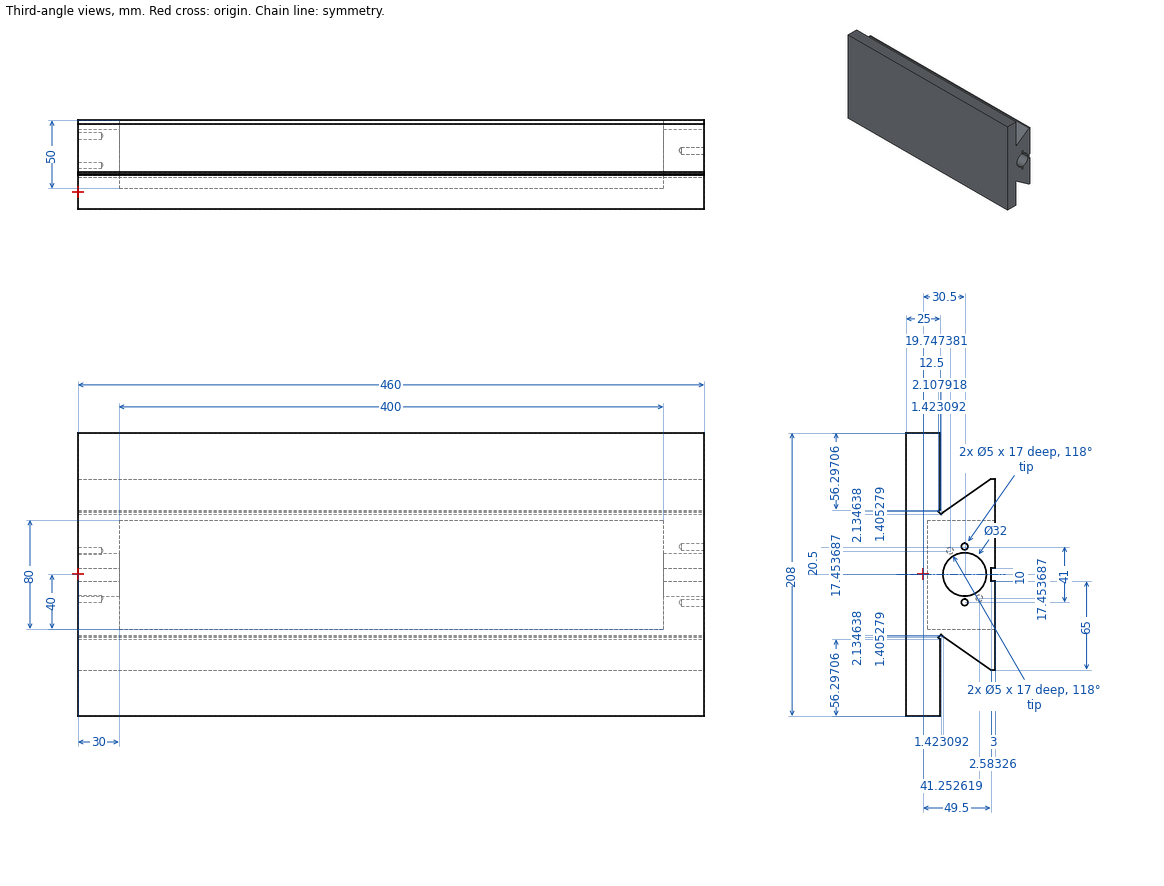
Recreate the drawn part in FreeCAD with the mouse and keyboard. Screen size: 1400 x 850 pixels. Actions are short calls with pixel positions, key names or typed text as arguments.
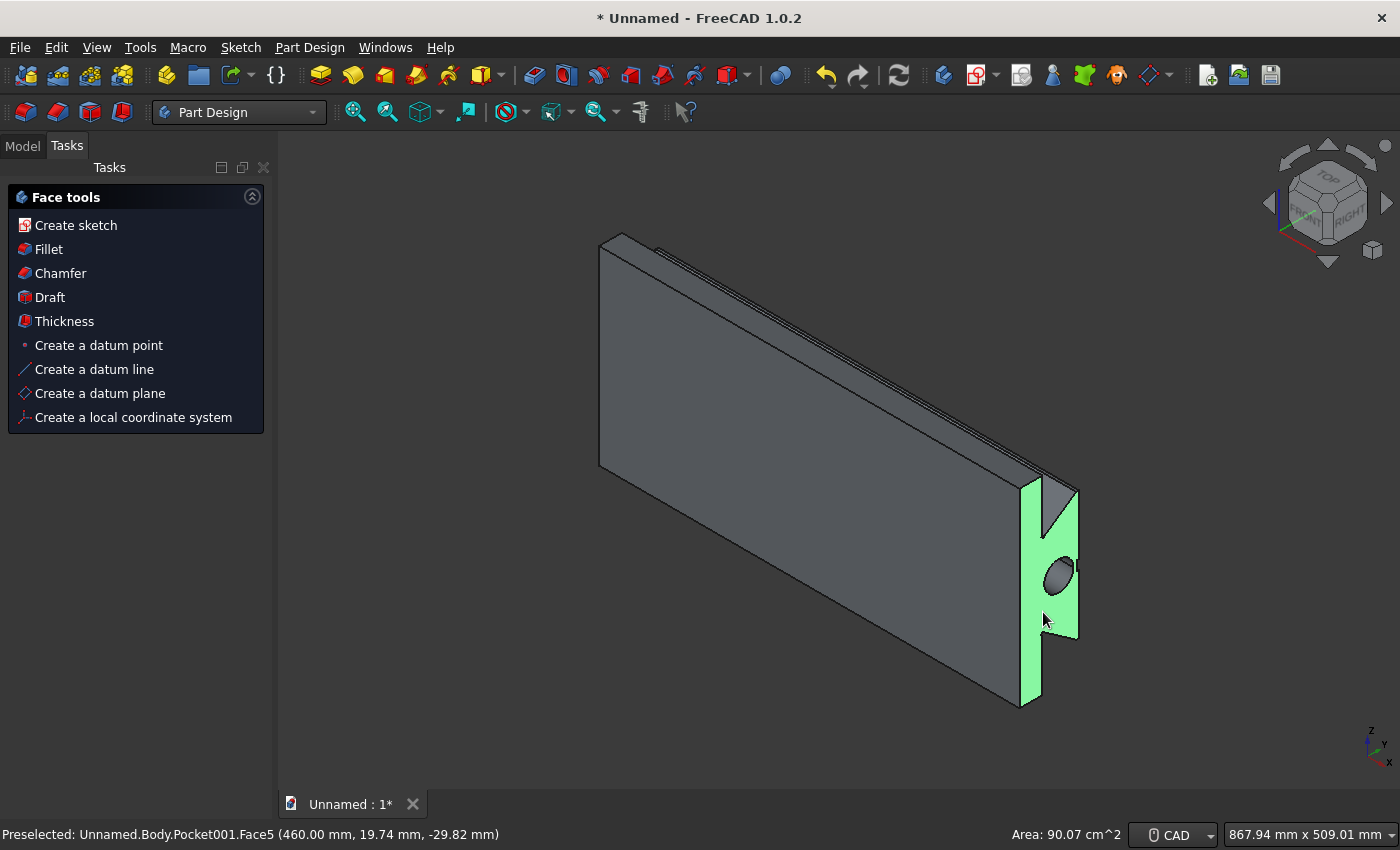
click(976, 76)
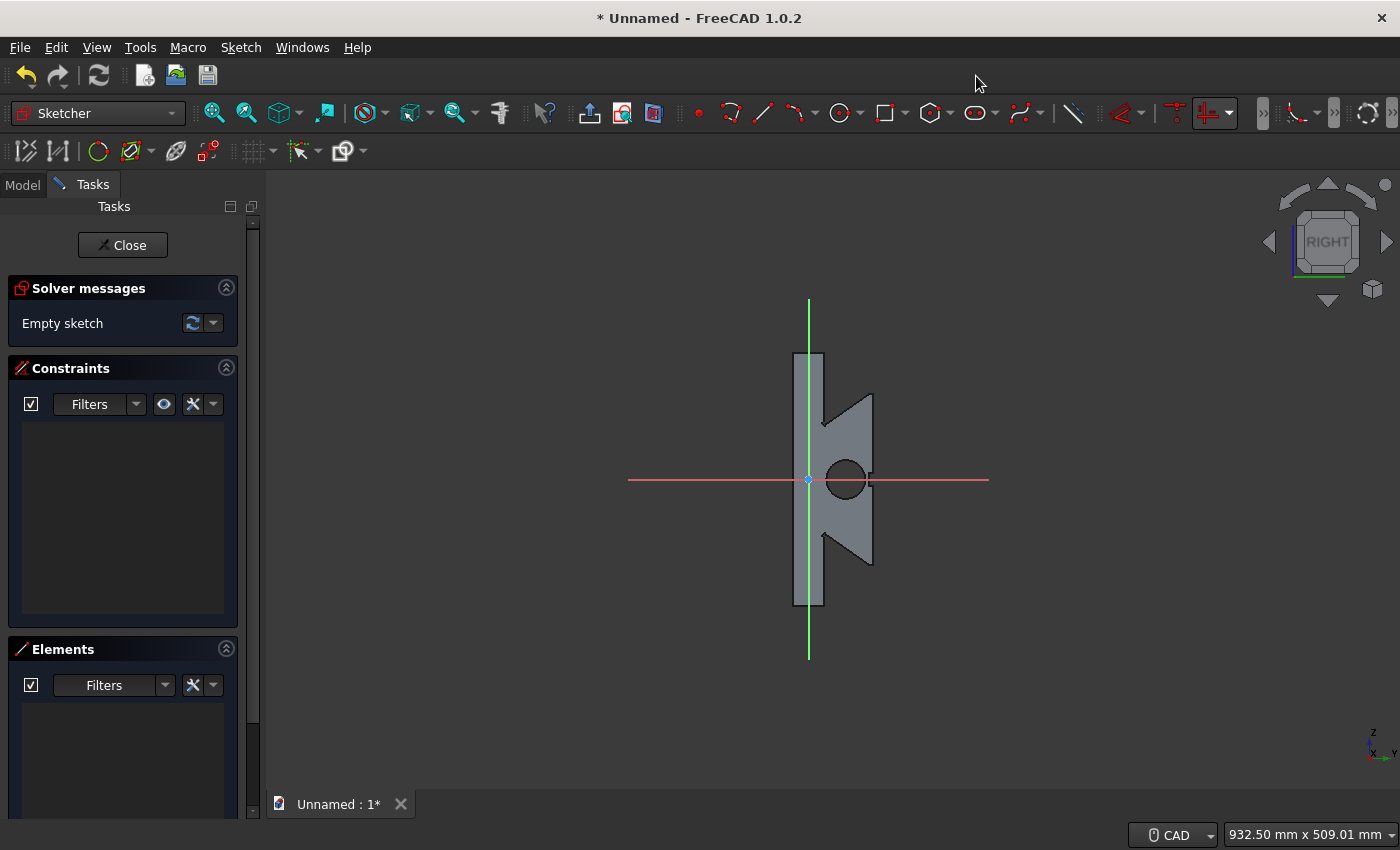
scroll(839, 480, up, 10)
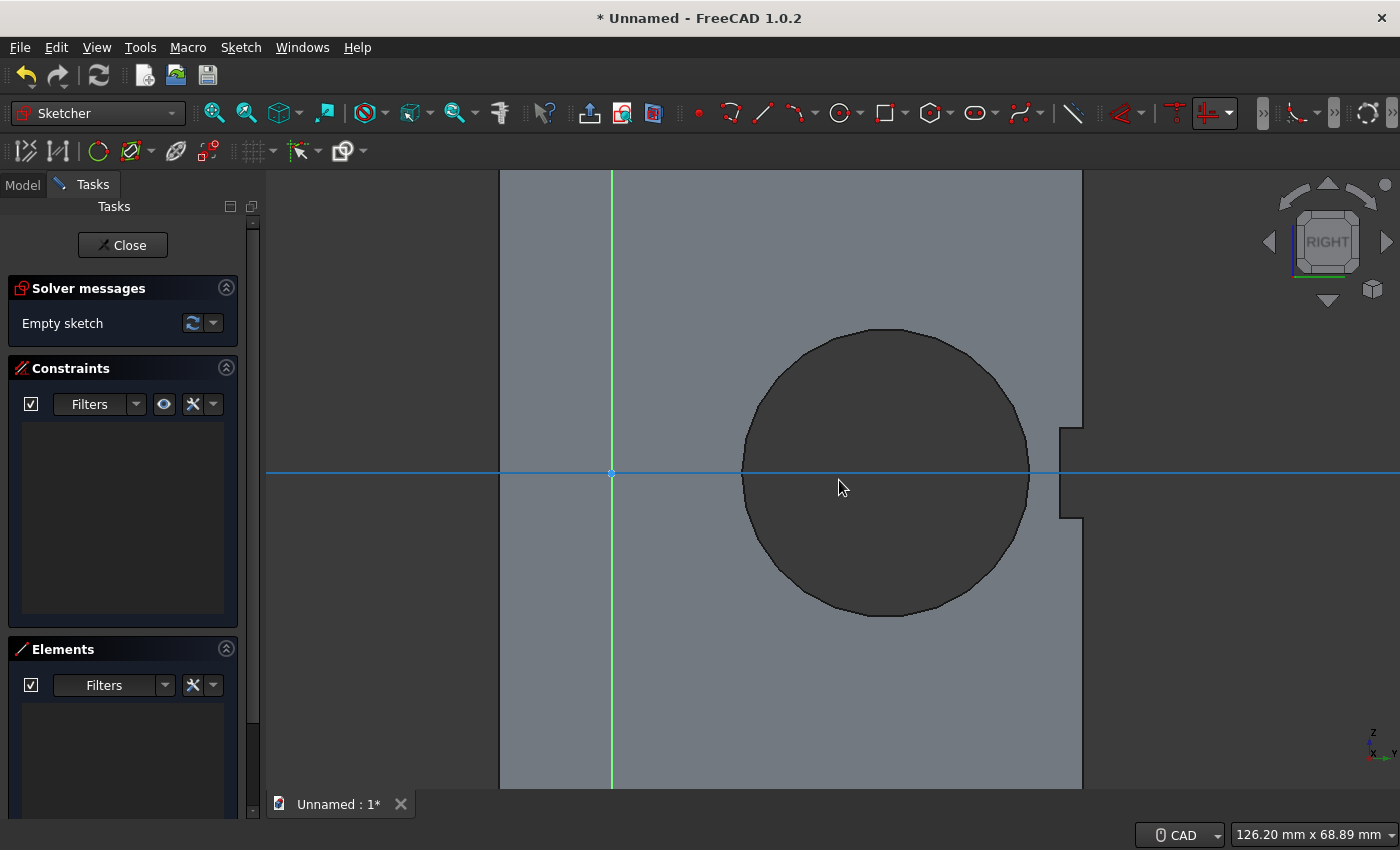
click(840, 114)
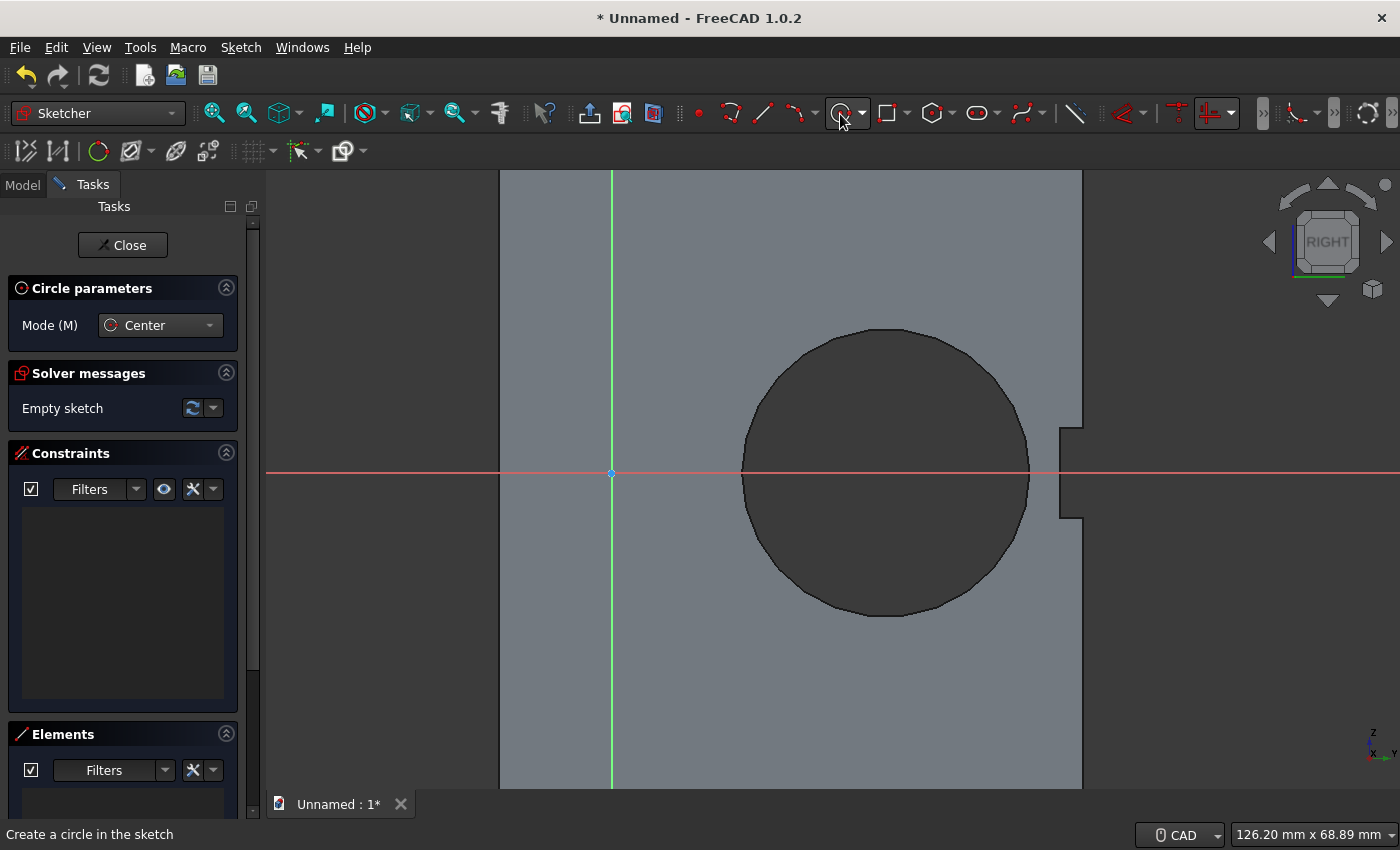
click(886, 289)
move(902, 273)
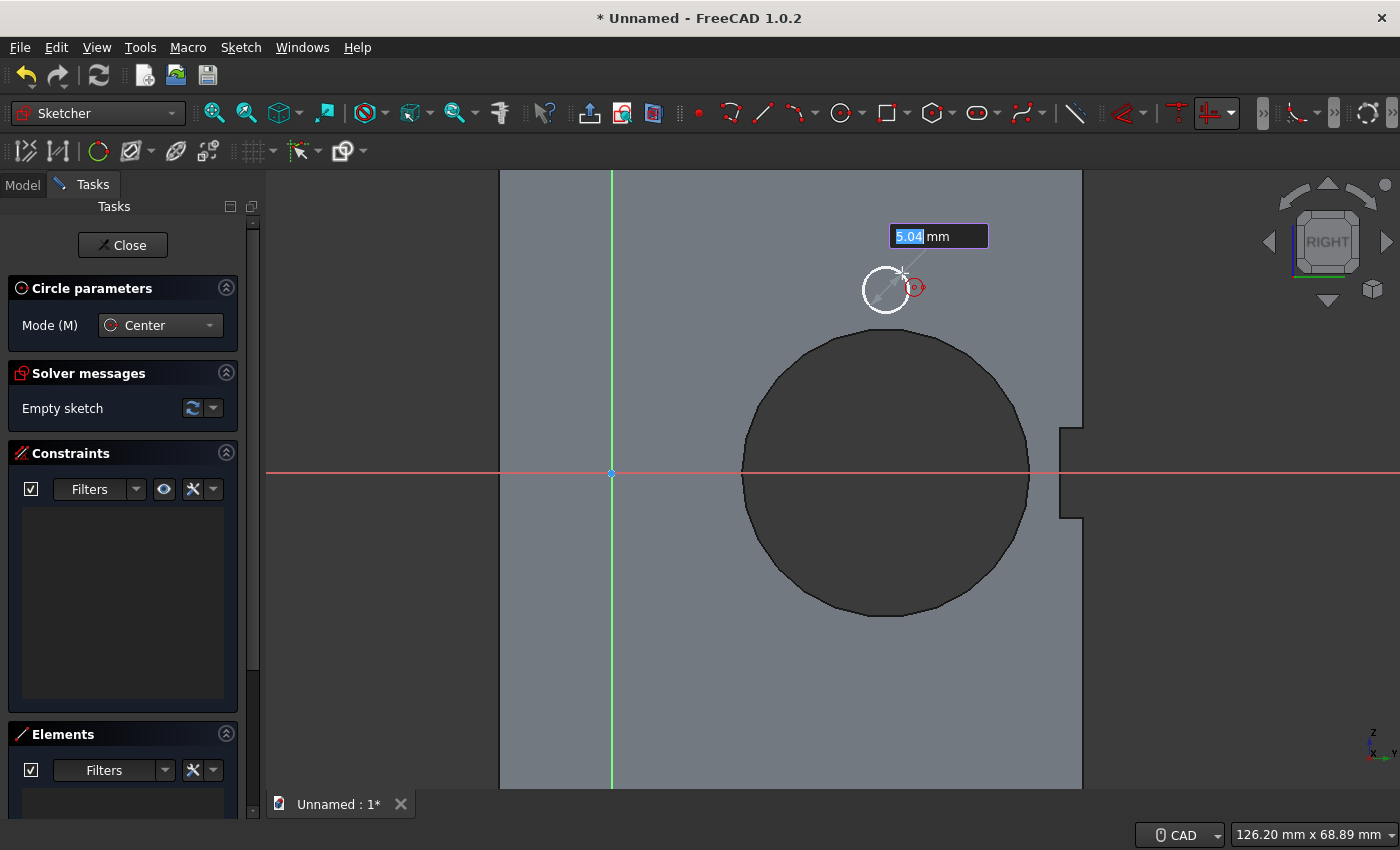
text(5)
key(Return)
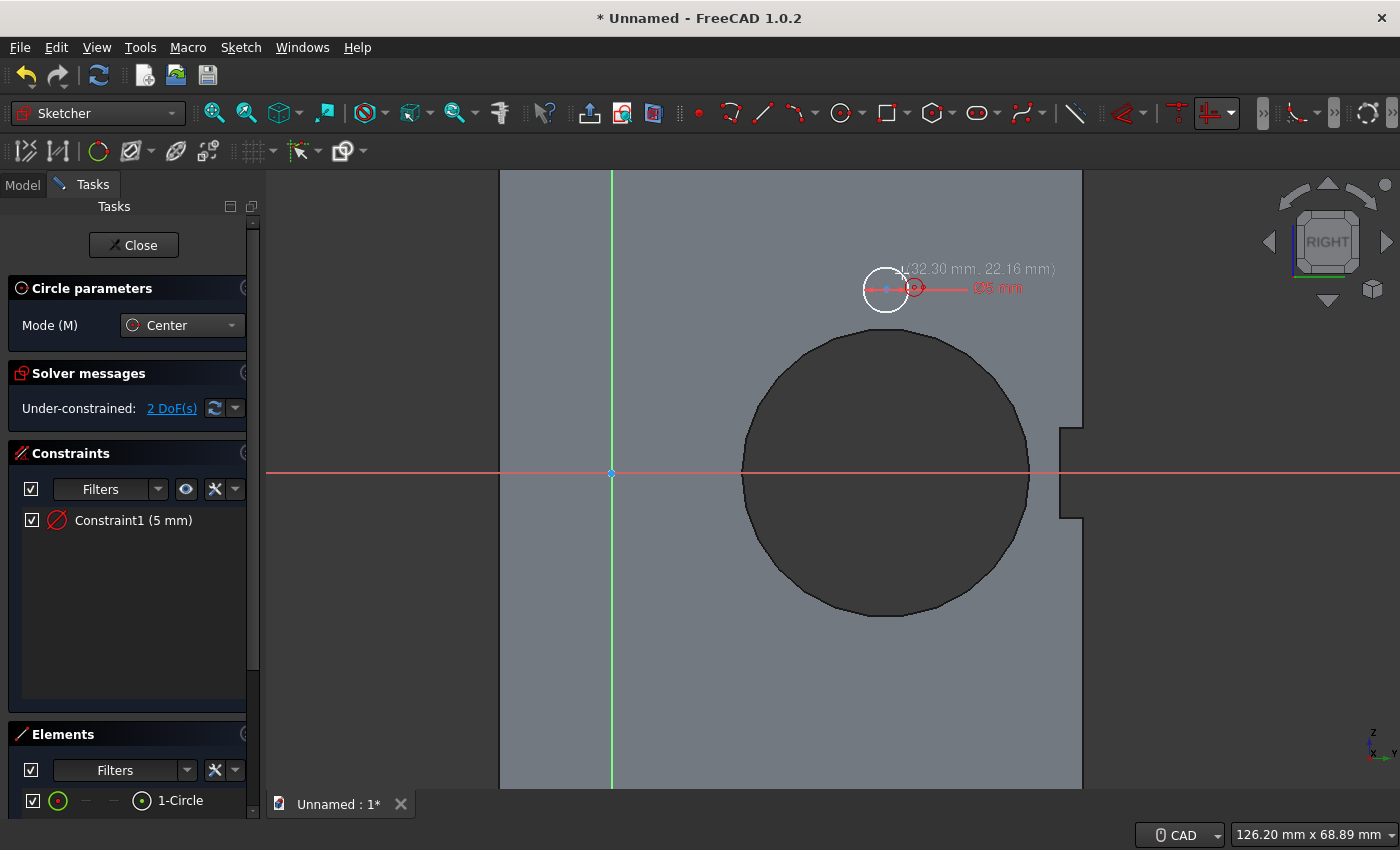
click(886, 657)
move(902, 641)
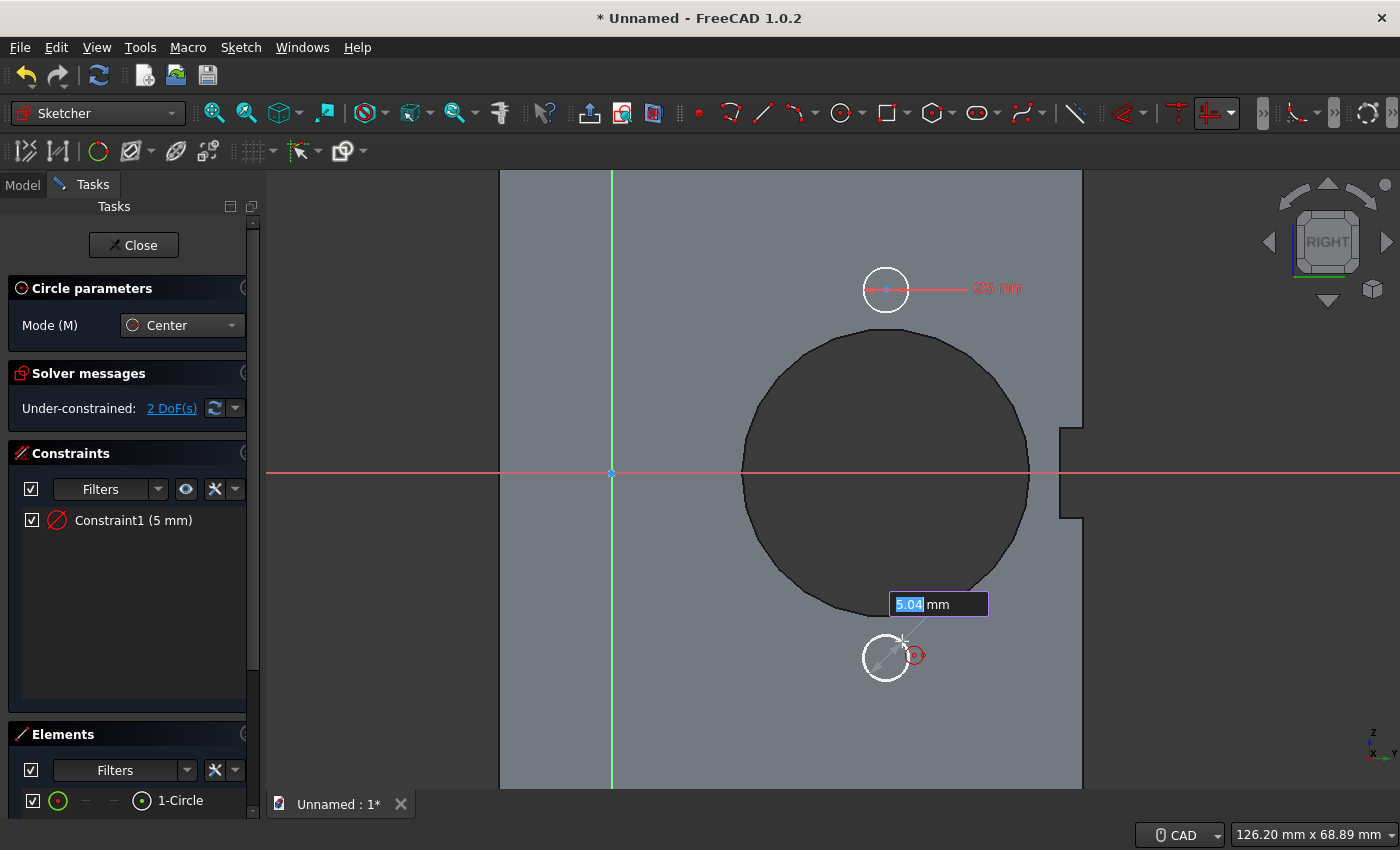
text(5)
key(Return)
key(Escape)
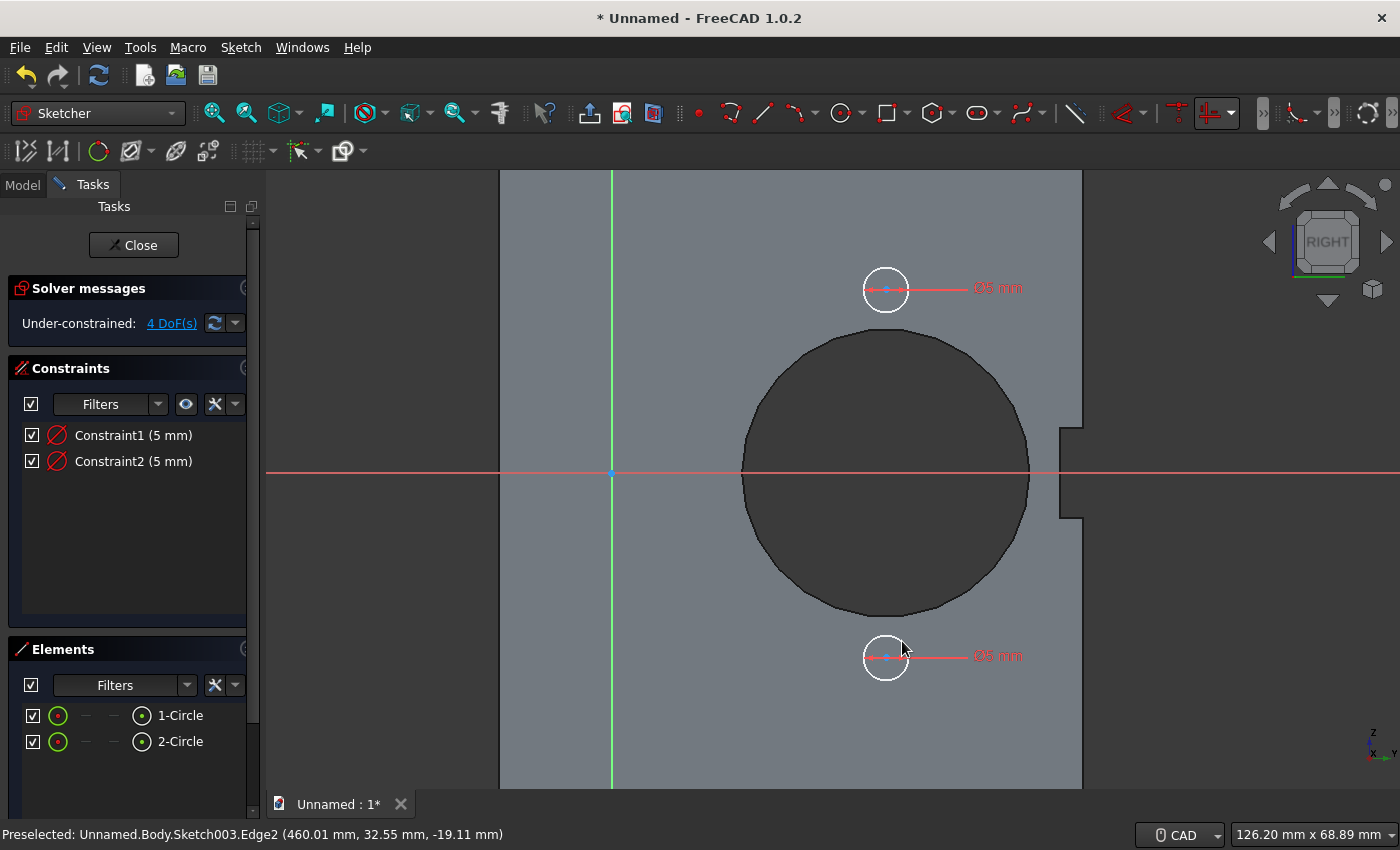
click(886, 290)